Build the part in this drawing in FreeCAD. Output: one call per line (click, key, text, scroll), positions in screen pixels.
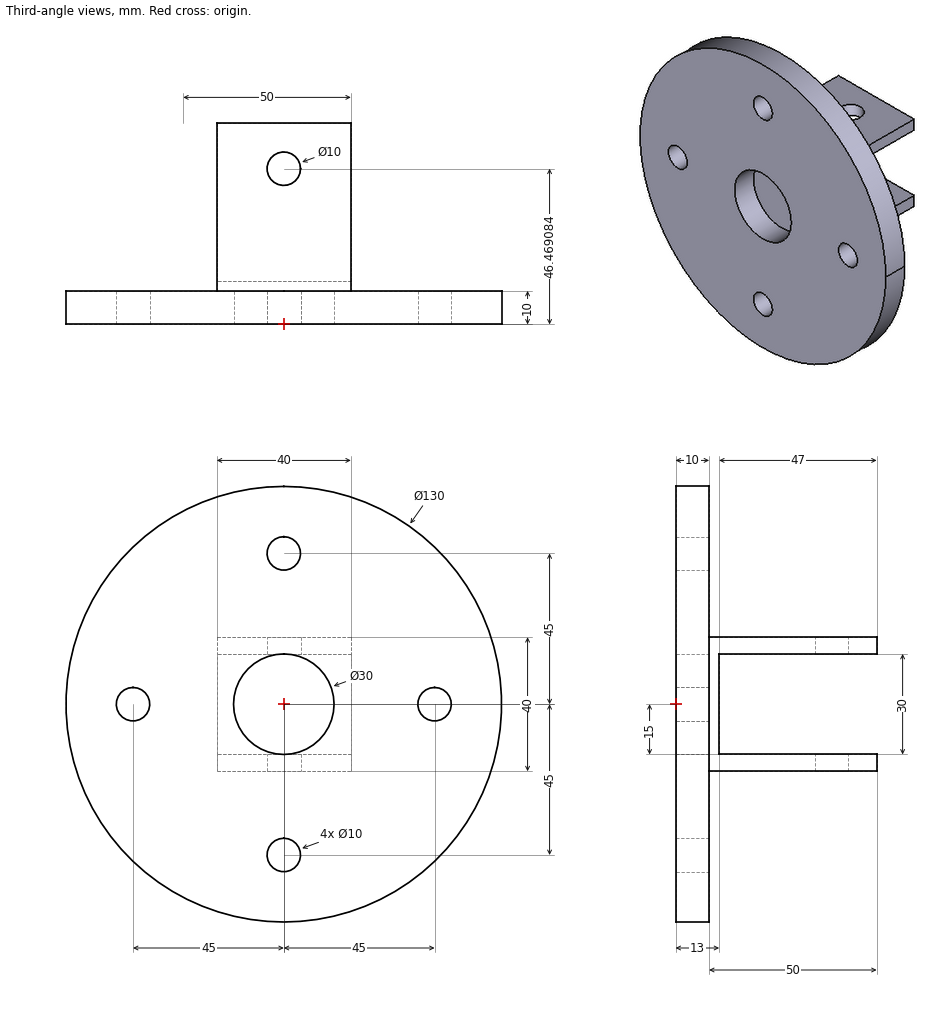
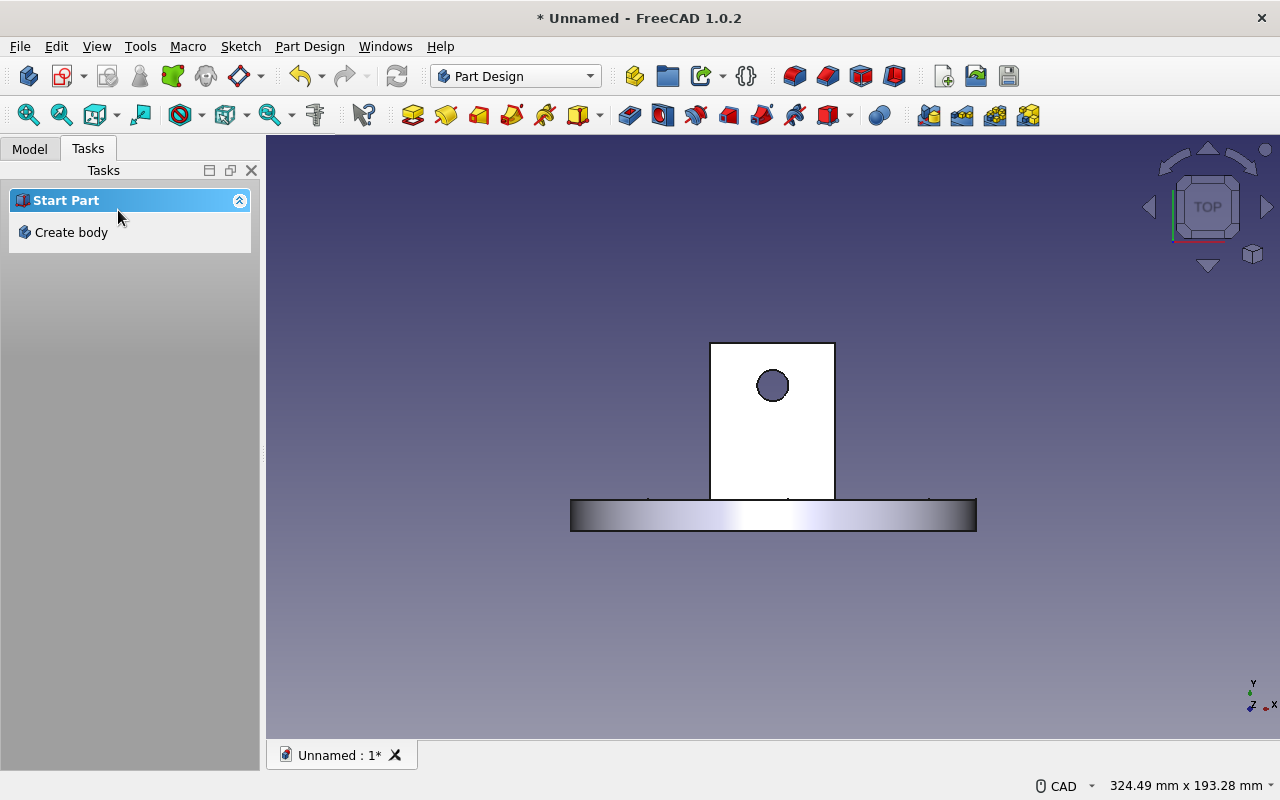
key(0)